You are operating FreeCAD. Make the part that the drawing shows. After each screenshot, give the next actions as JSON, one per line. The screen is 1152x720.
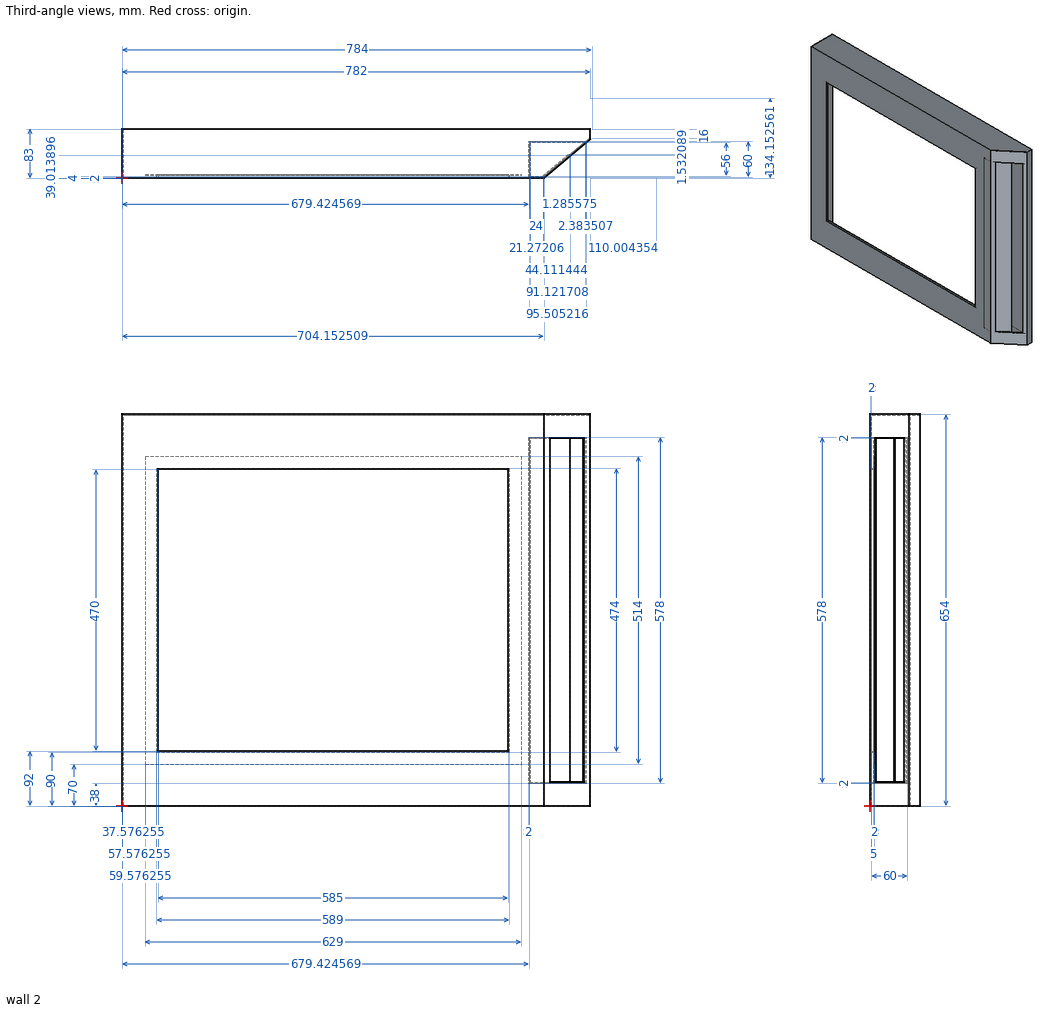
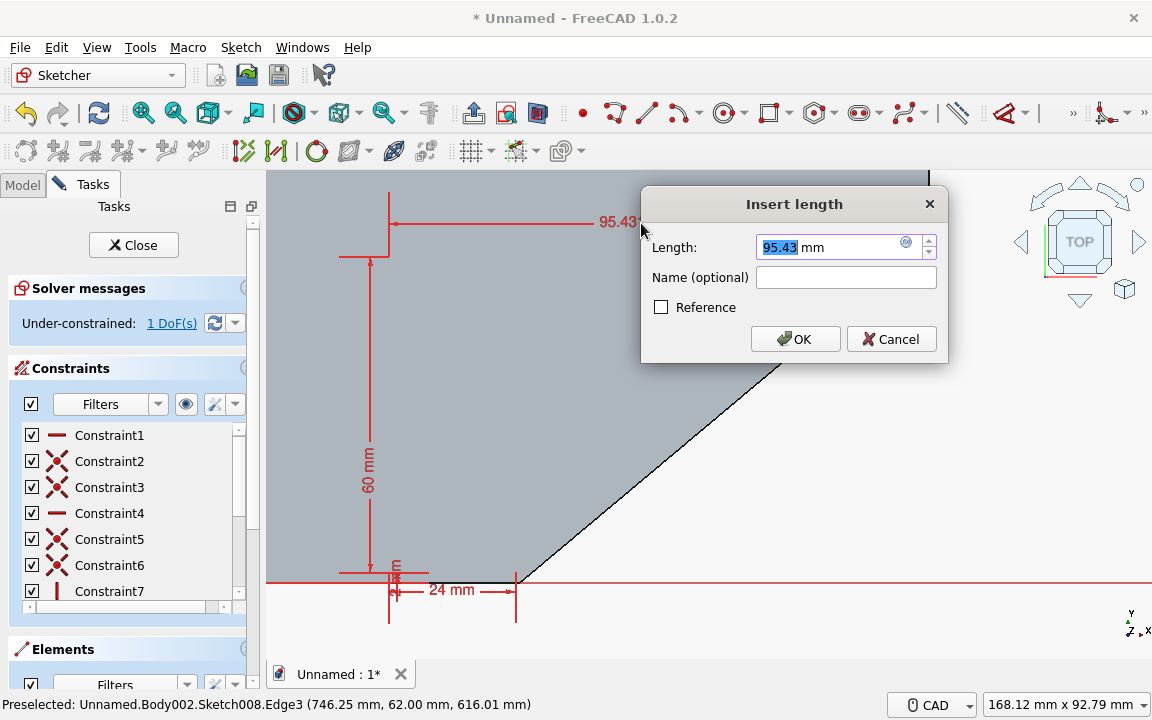
{"action": "type", "text": "95.505216"}
{"action": "key", "text": "Return"}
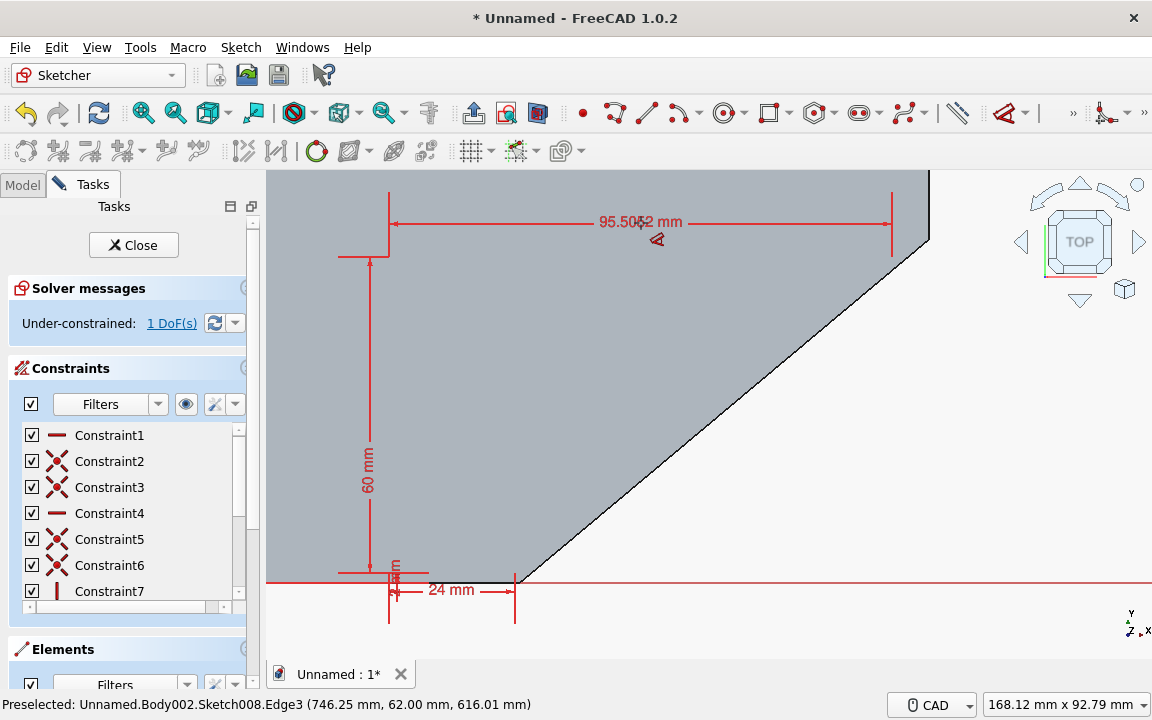
{"action": "left_click", "coordinate": [389, 573]}
{"action": "left_click", "coordinate": [341, 617]}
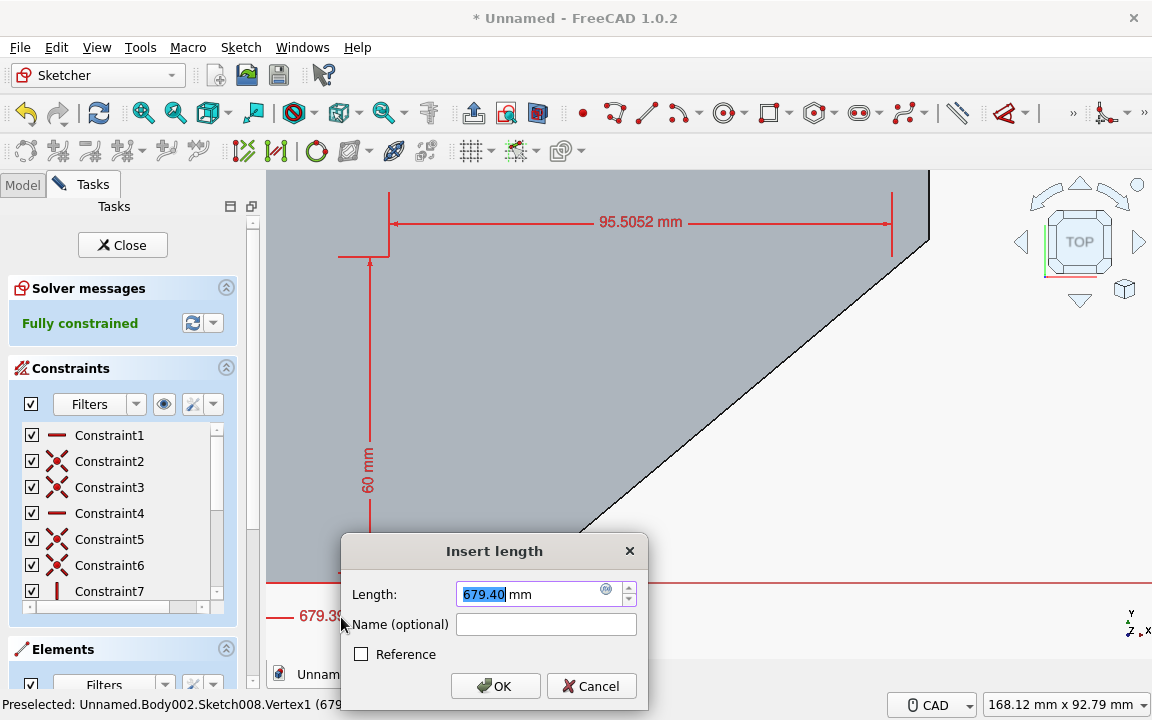
{"action": "type", "text": "679.424569"}
{"action": "key", "text": "Return"}
{"action": "key", "text": "Escape"}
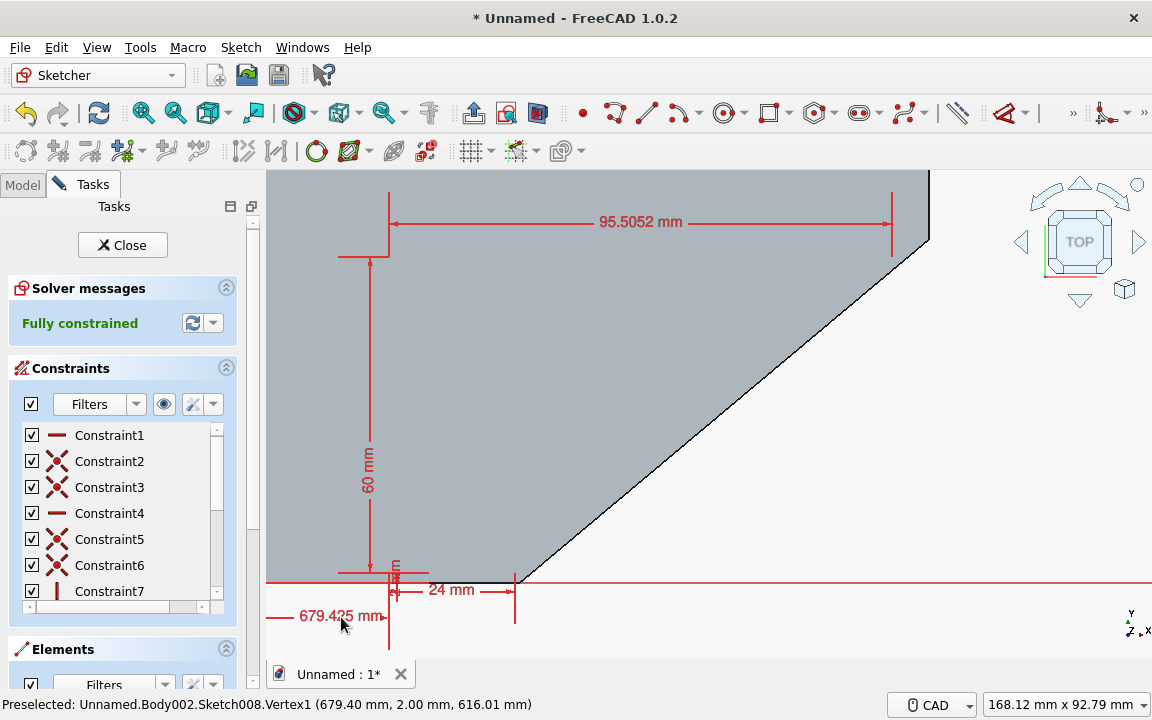
{"action": "left_click", "coordinate": [123, 245]}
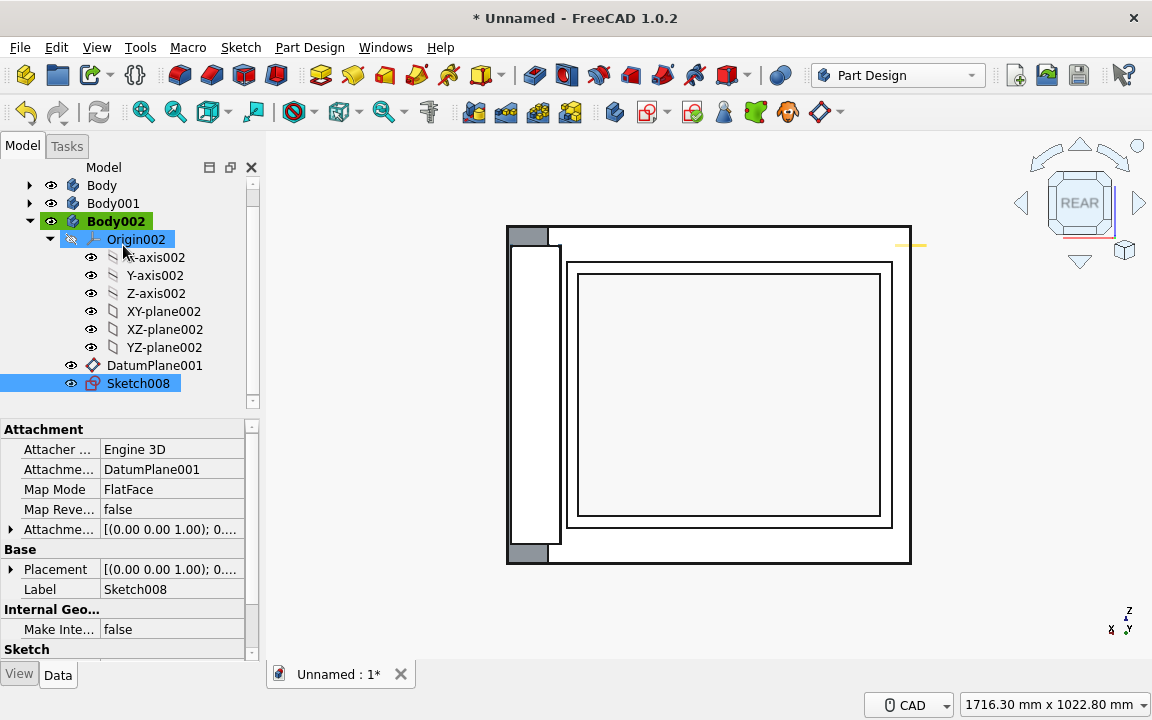
{"action": "left_click", "coordinate": [322, 76]}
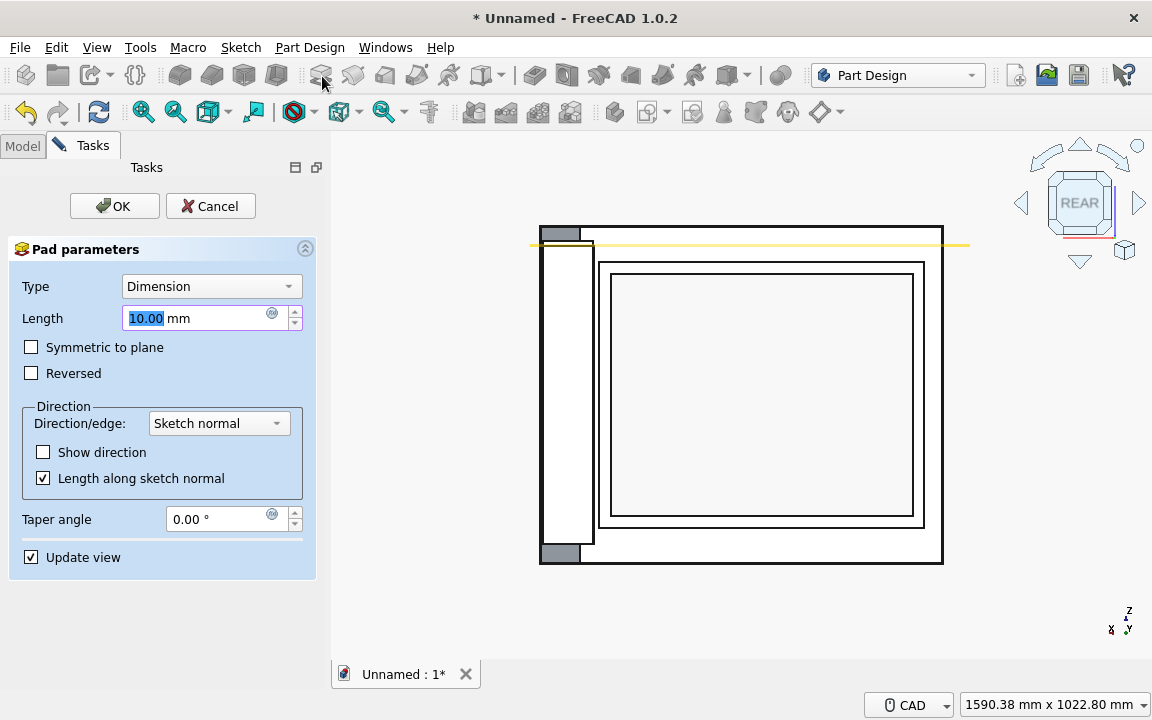
{"action": "type", "text": "2"}
{"action": "key", "text": "Tab"}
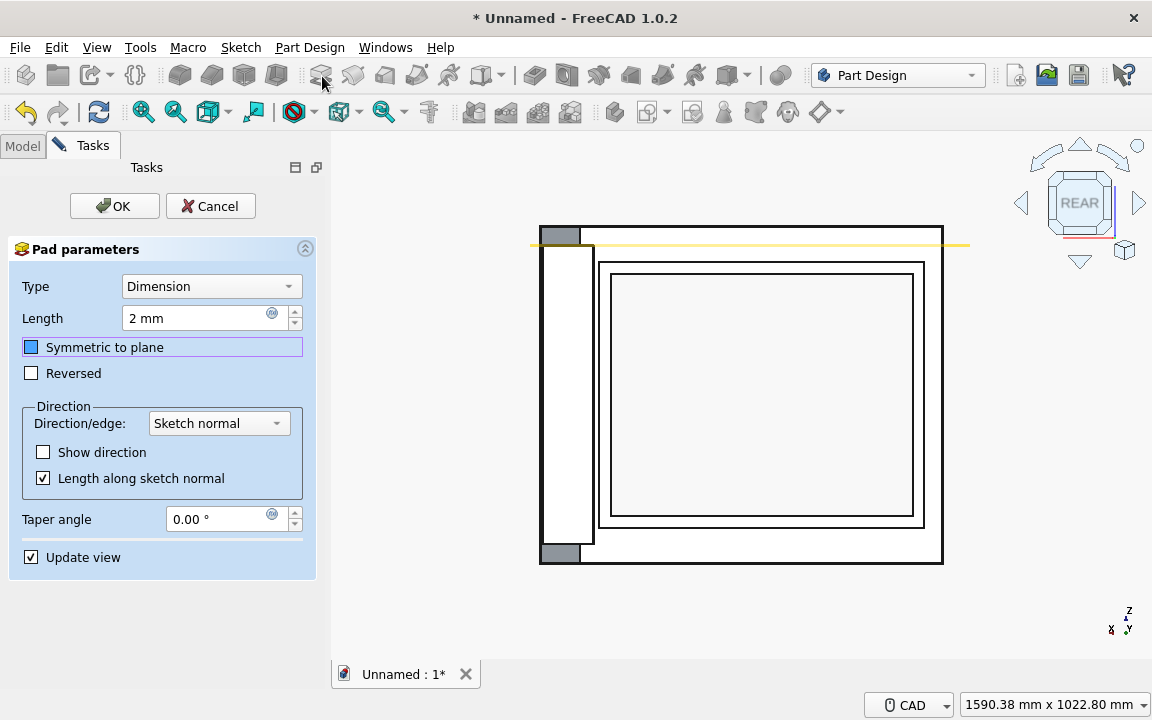
{"action": "left_click", "coordinate": [30, 373]}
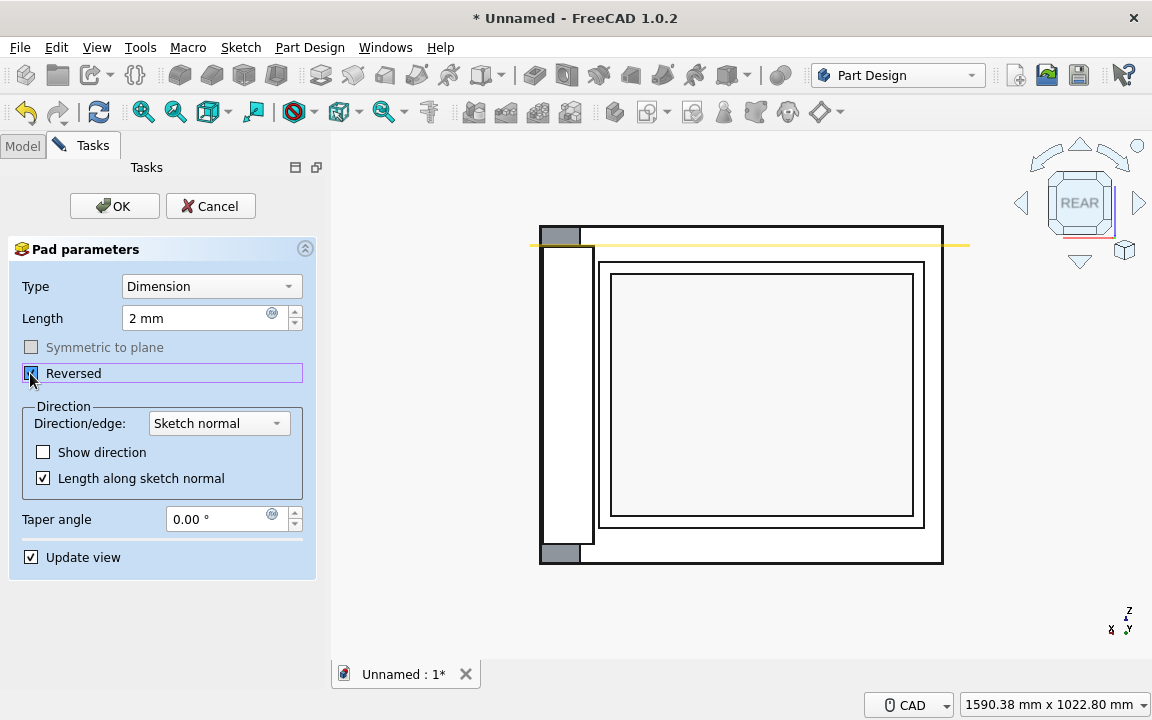
{"action": "left_click", "coordinate": [115, 206]}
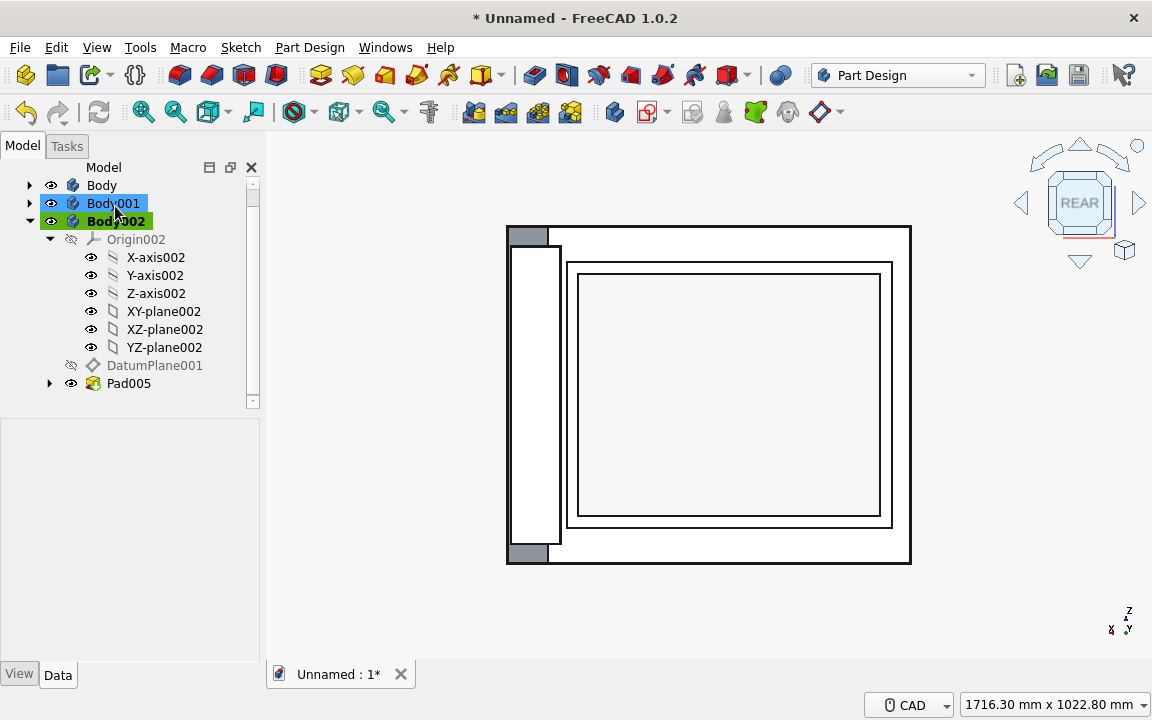
{"action": "left_click", "coordinate": [144, 112]}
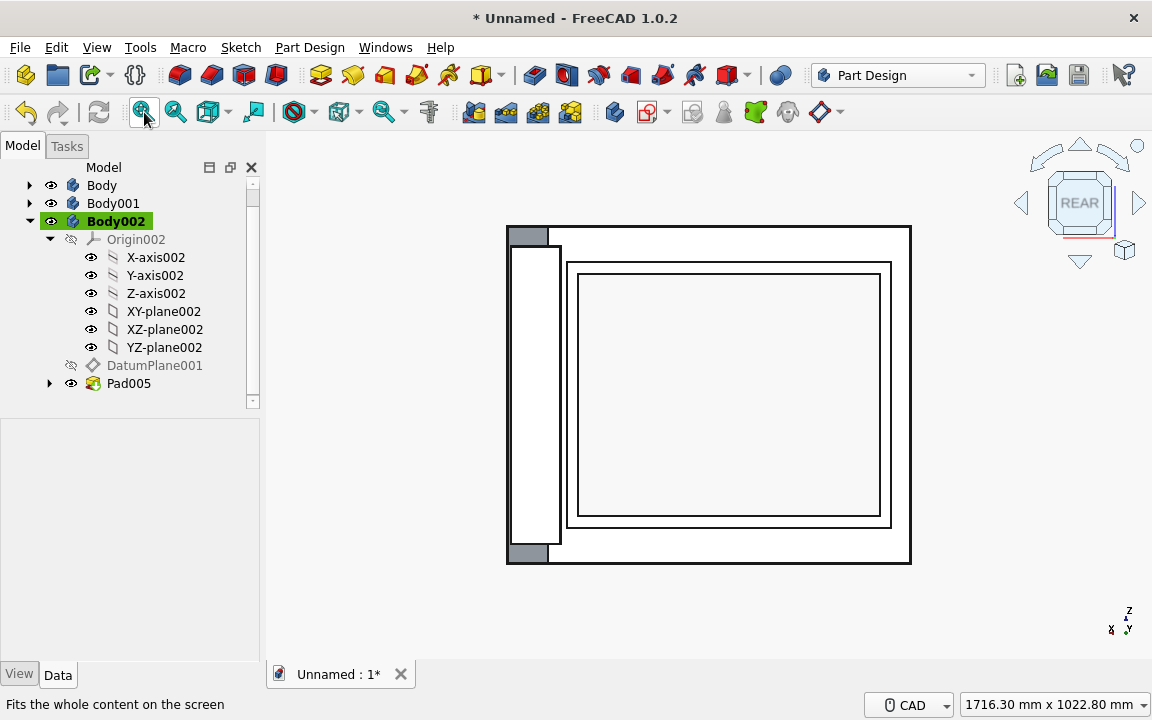
{"action": "left_click", "coordinate": [616, 112]}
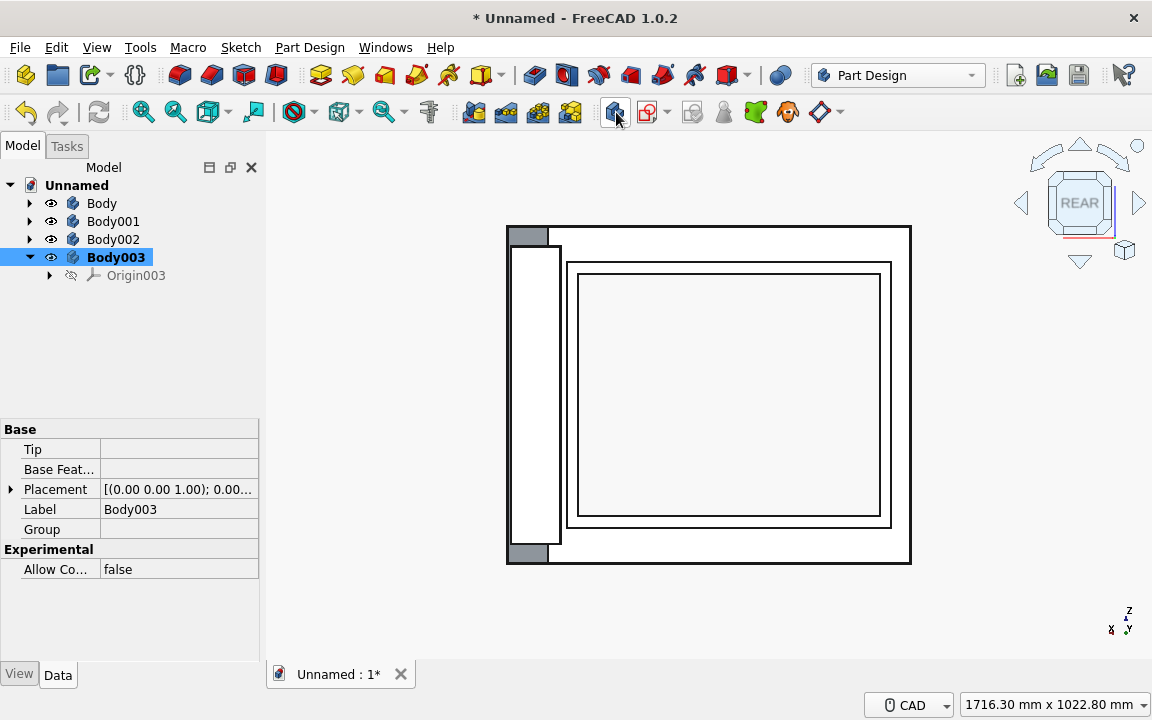
{"action": "left_click", "coordinate": [50, 275]}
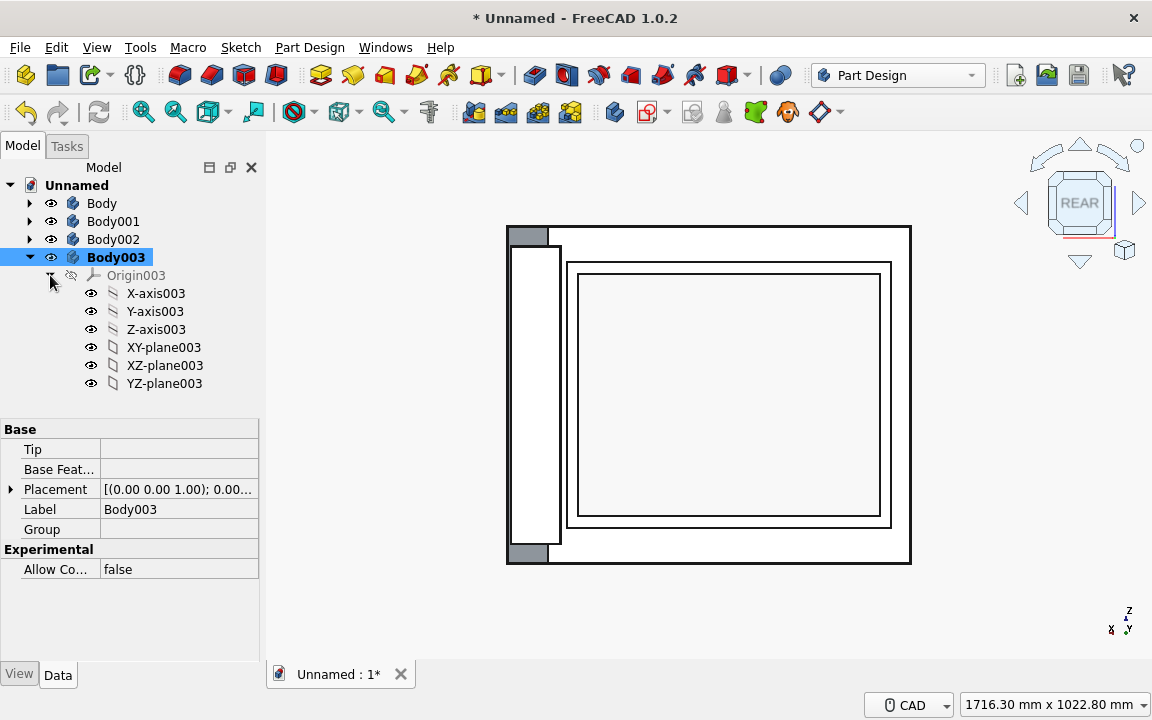
{"action": "left_click", "coordinate": [136, 347]}